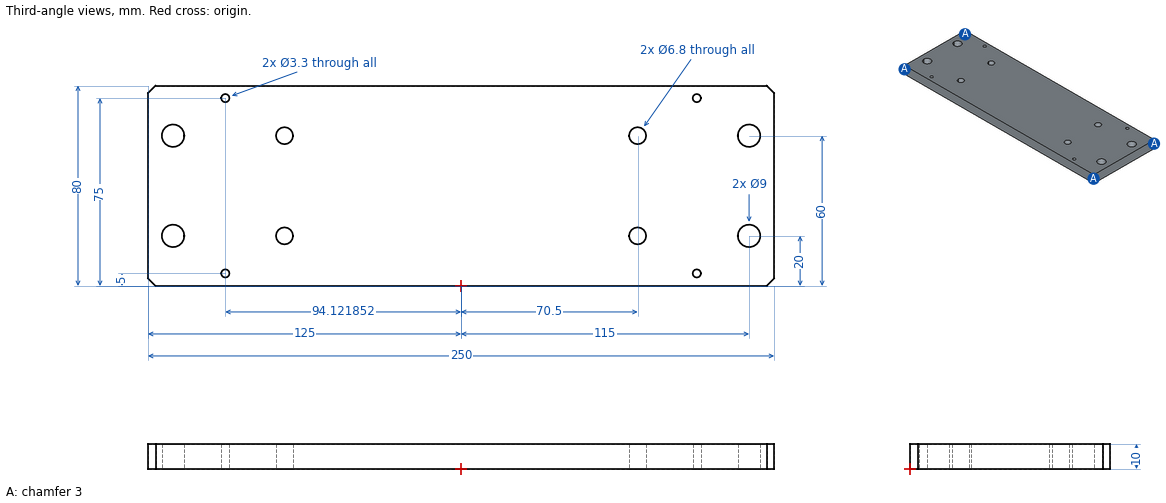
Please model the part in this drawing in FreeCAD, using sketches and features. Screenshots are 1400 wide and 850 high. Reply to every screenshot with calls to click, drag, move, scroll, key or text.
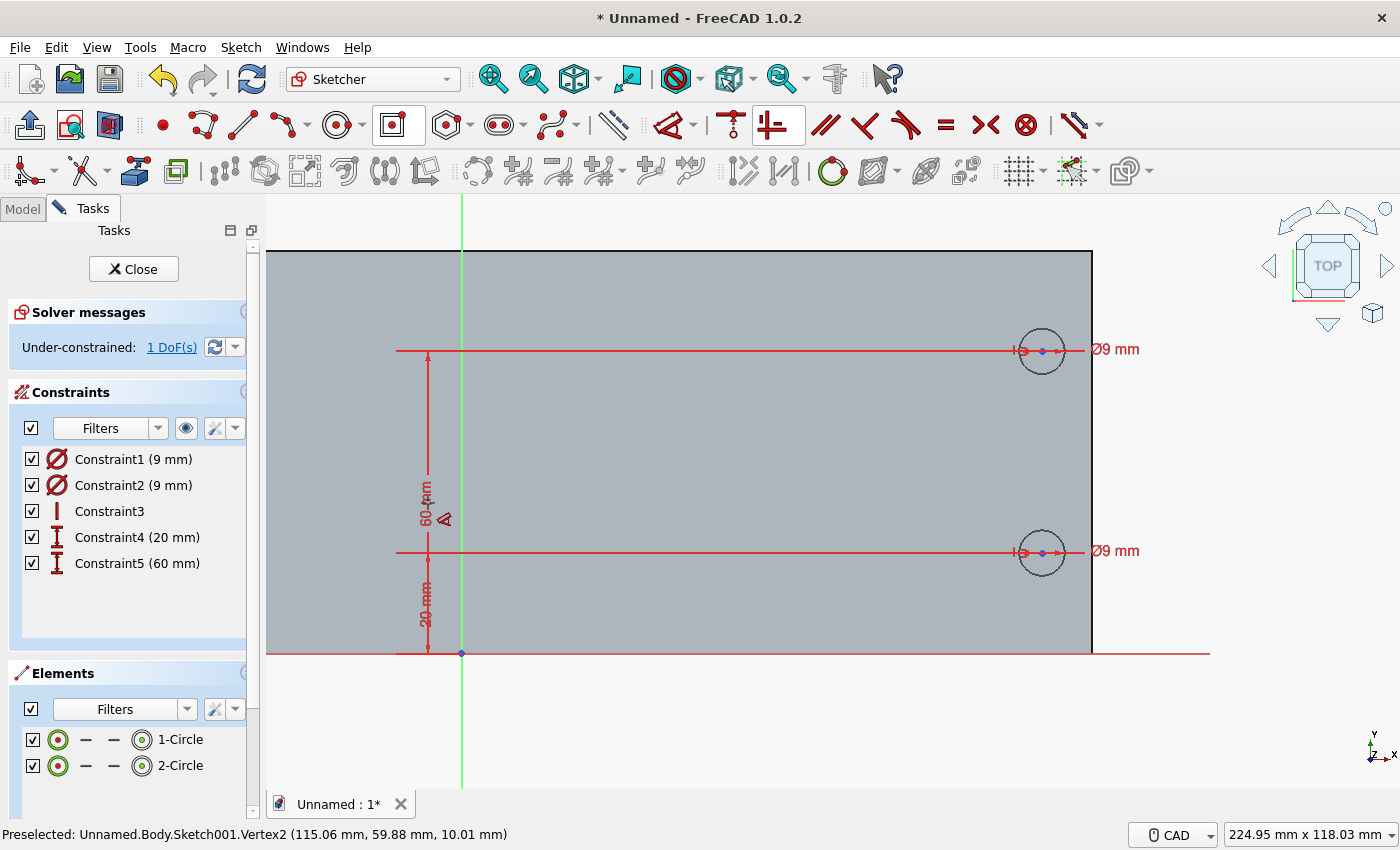
click(1042, 553)
click(752, 688)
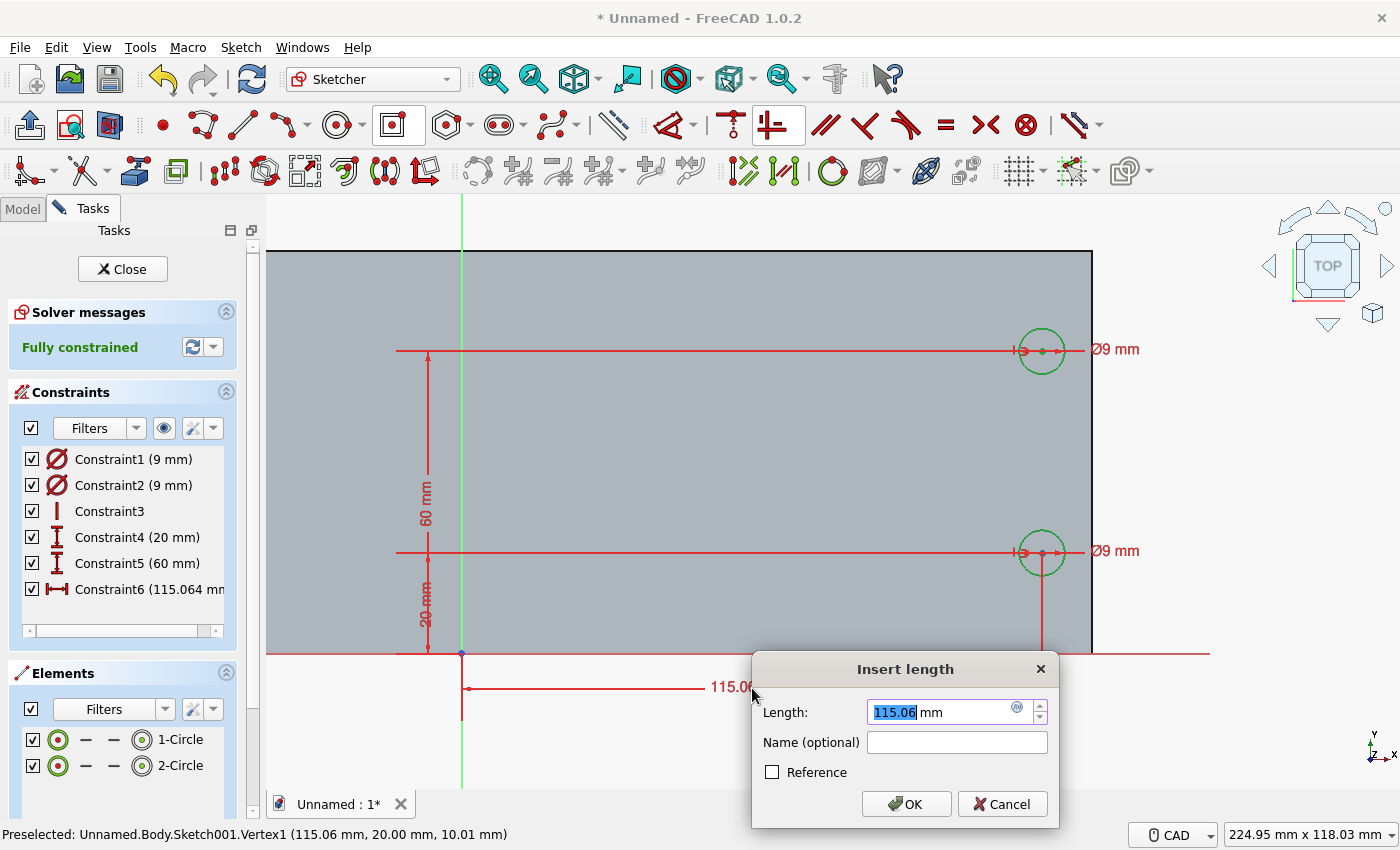
text(115)
key(Return)
key(Escape)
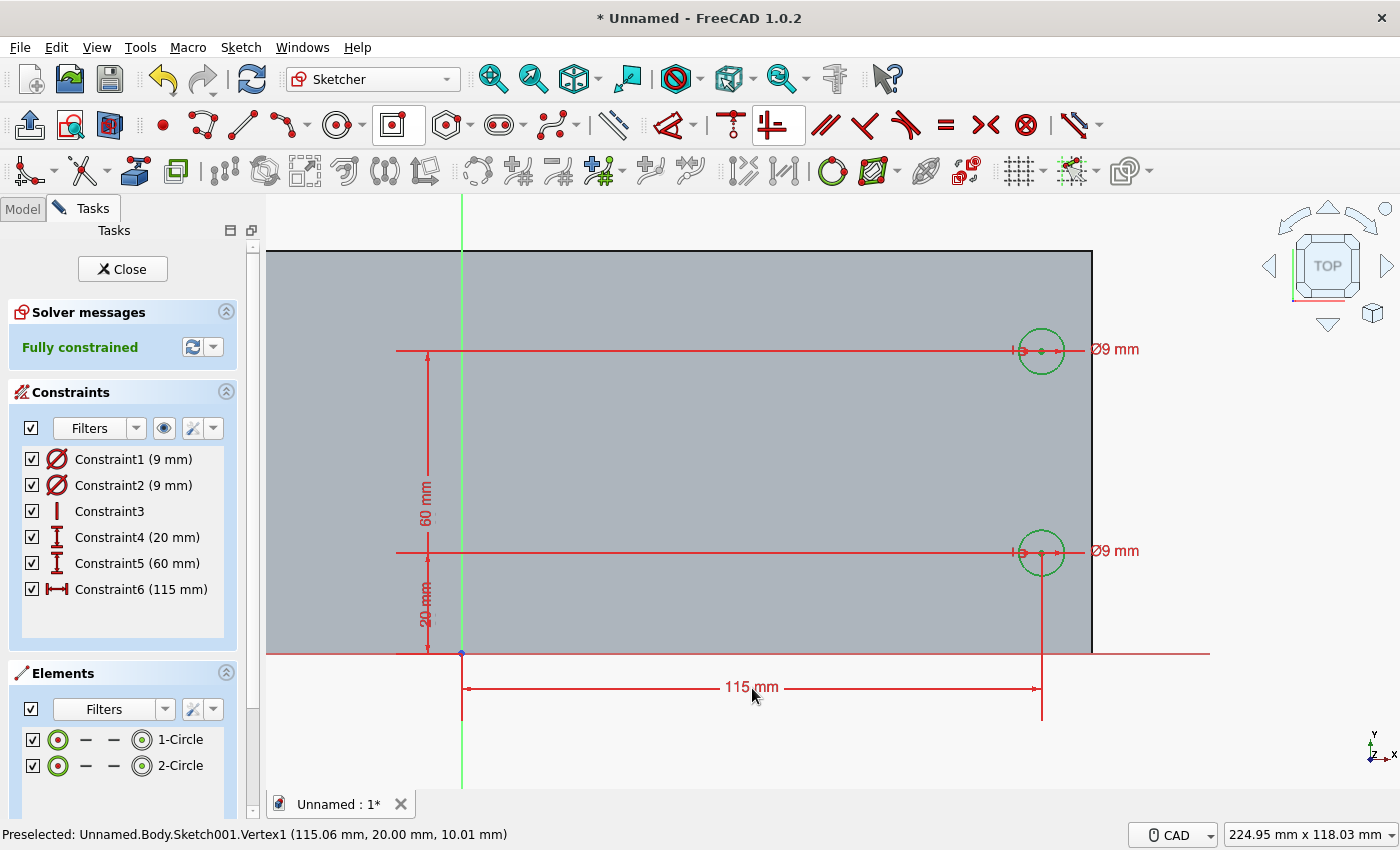
click(123, 269)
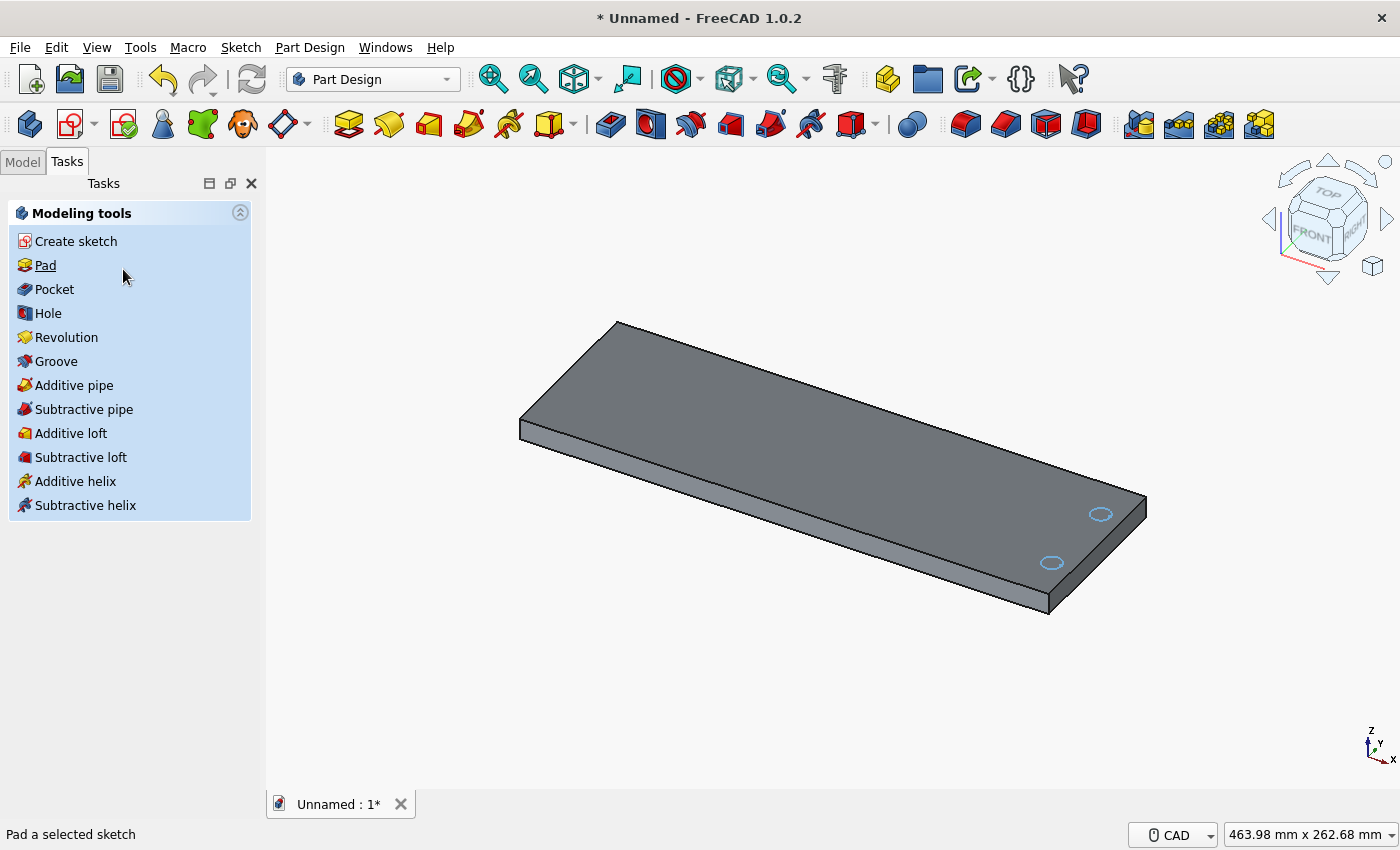
click(612, 124)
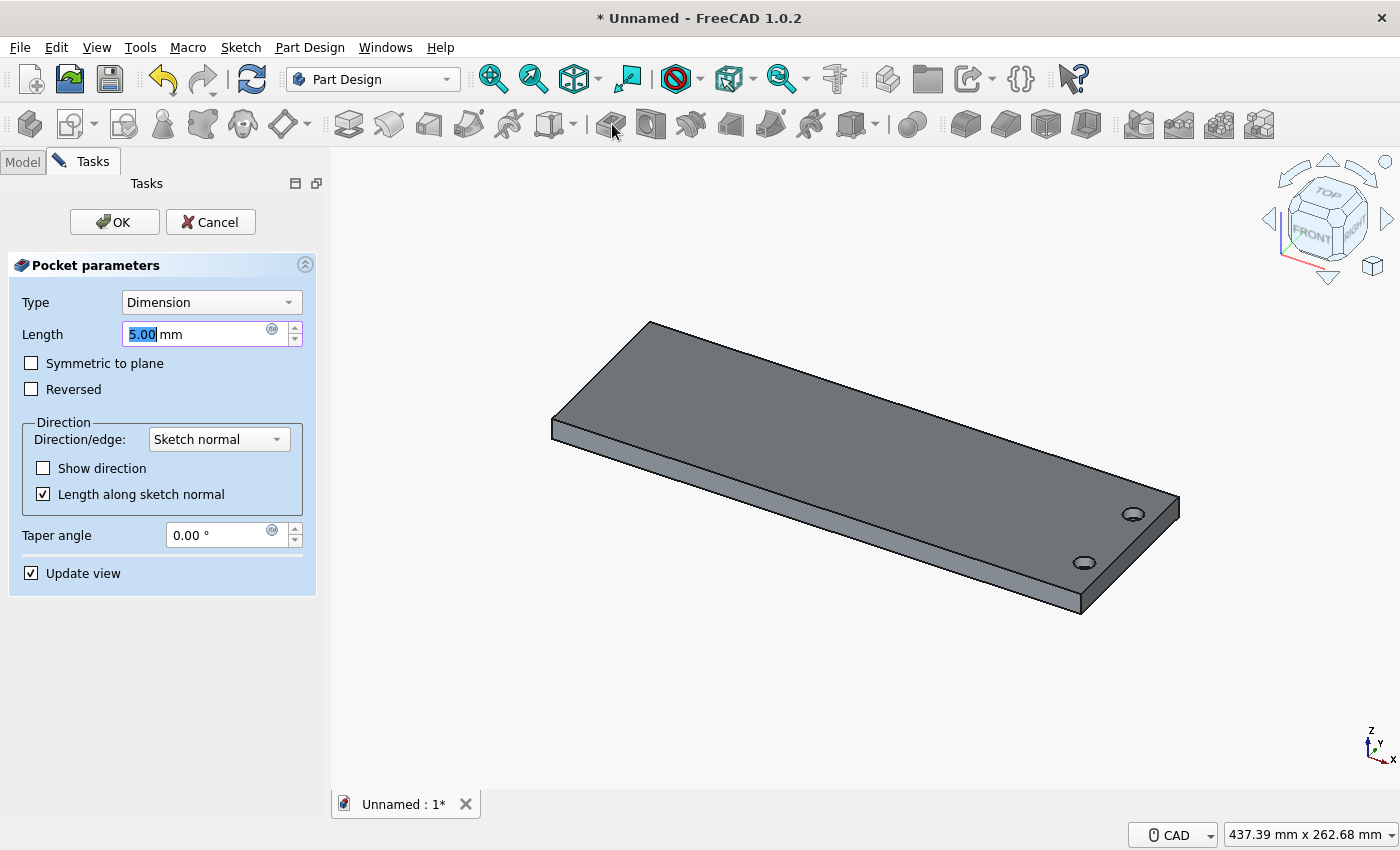
click(212, 302)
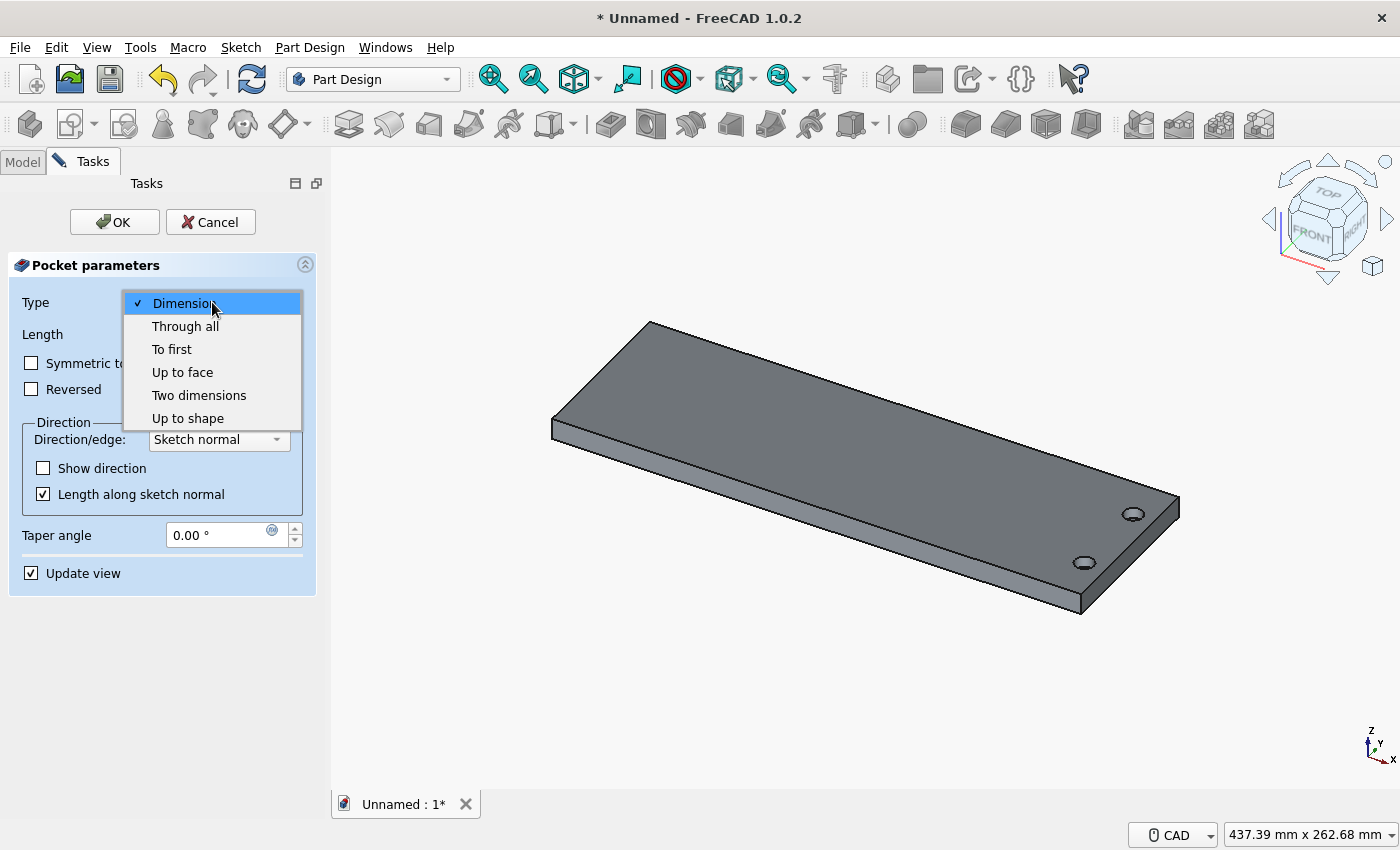
click(212, 326)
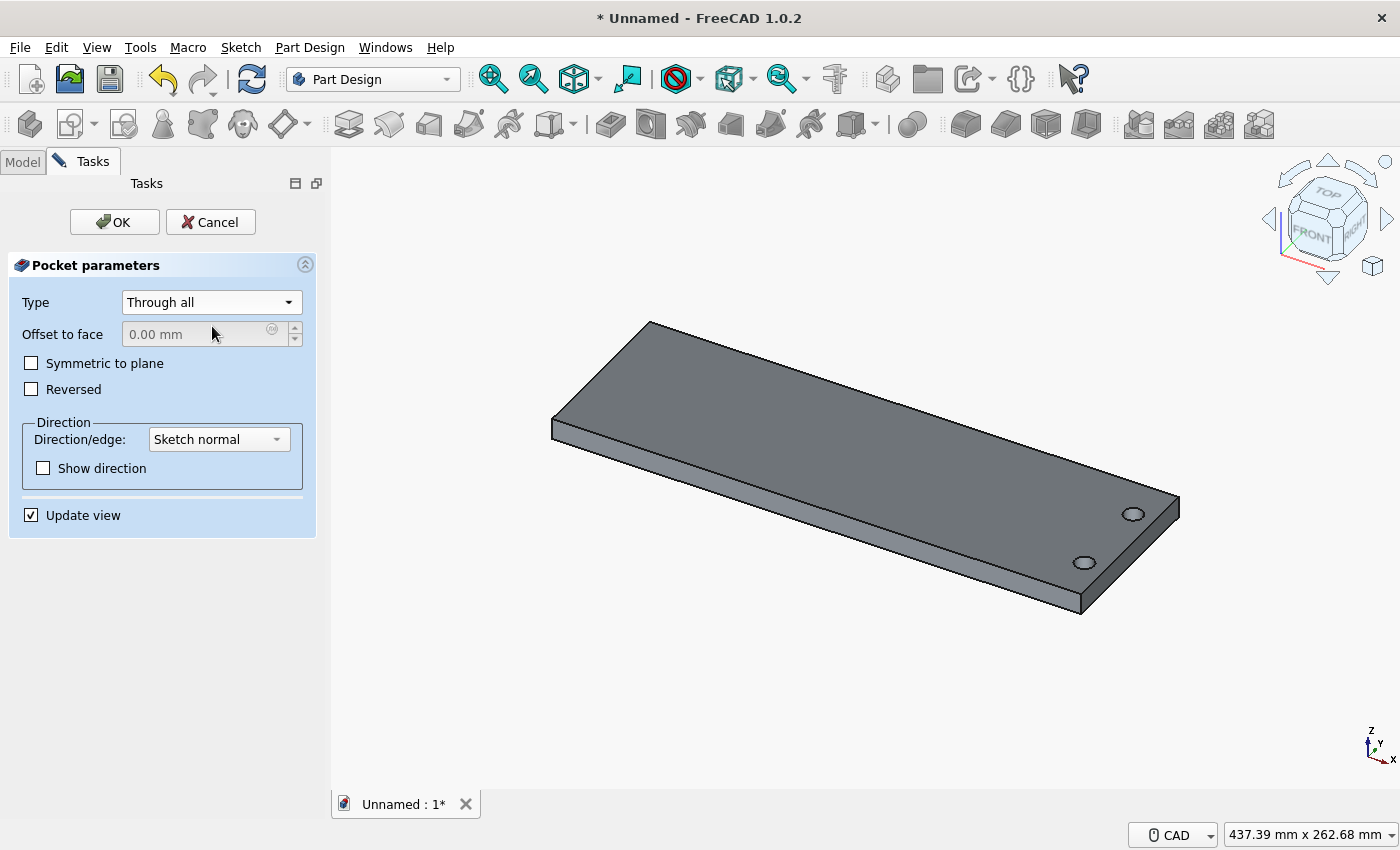
click(115, 222)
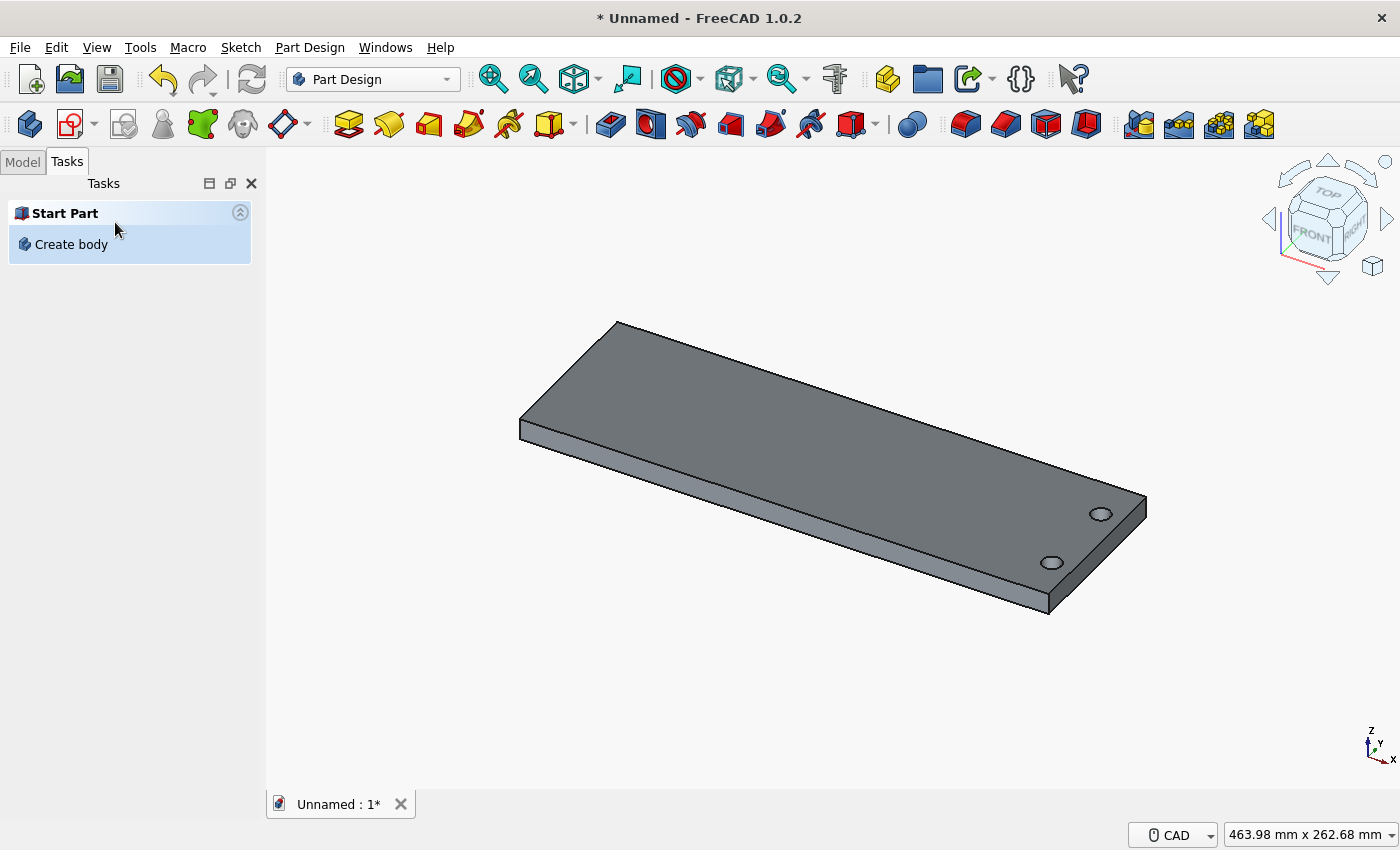
click(23, 161)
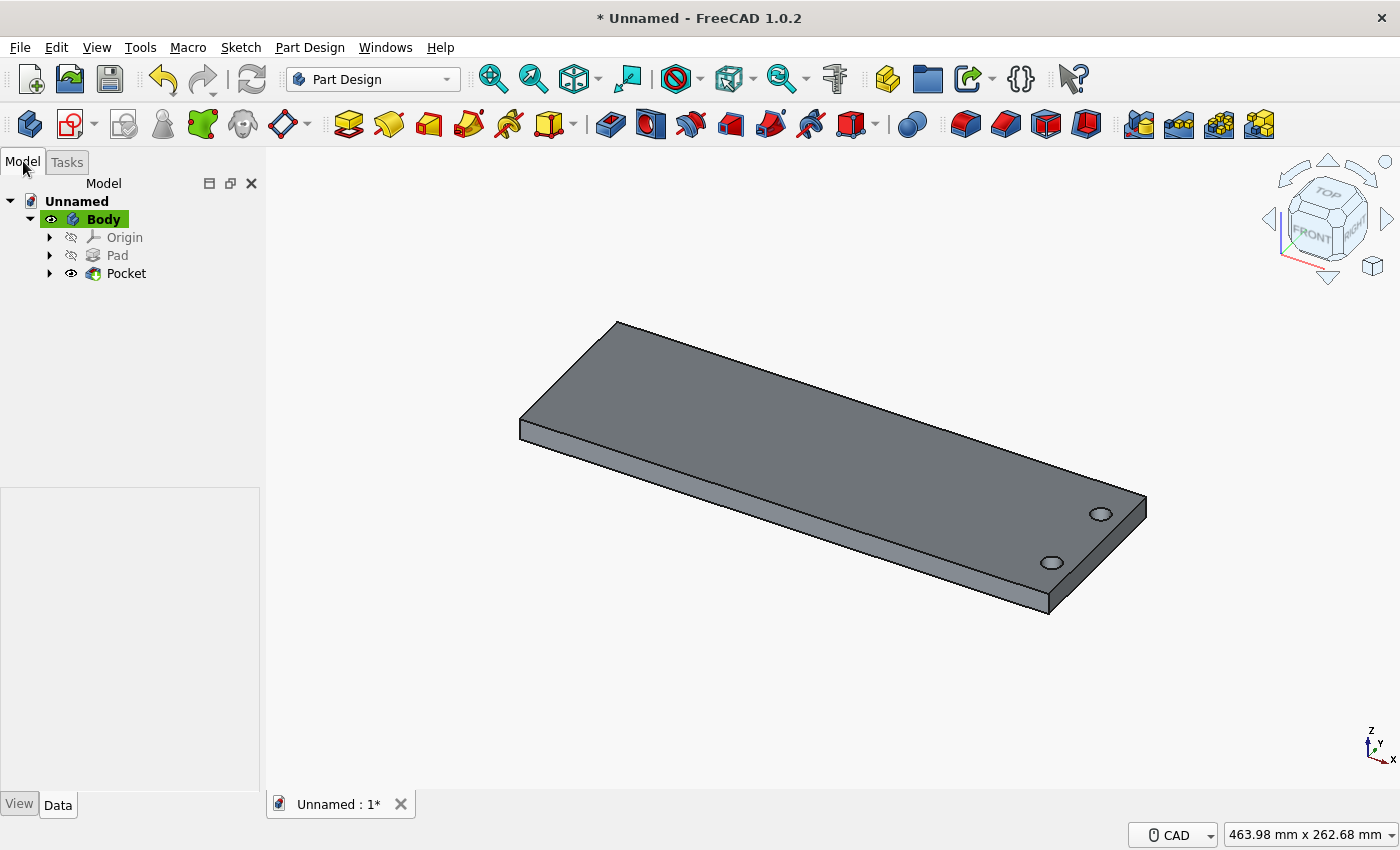
click(116, 273)